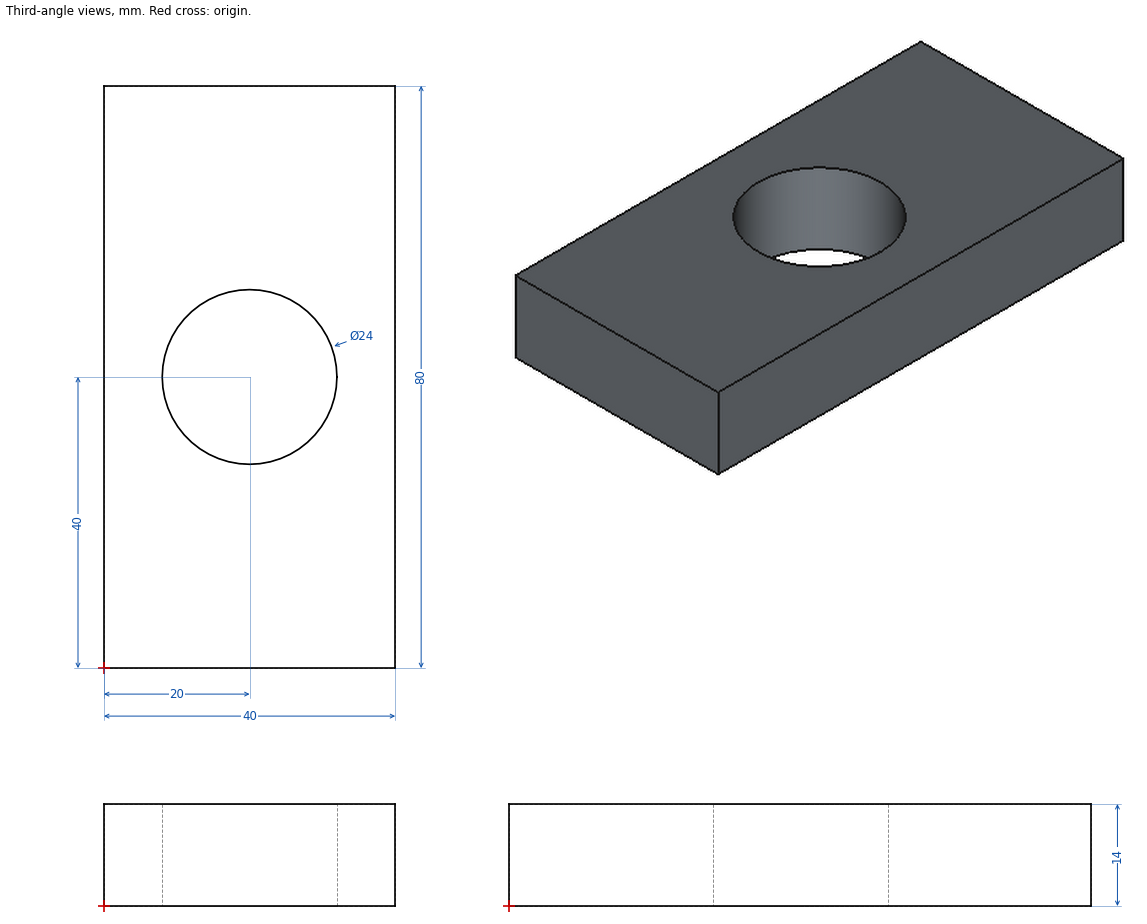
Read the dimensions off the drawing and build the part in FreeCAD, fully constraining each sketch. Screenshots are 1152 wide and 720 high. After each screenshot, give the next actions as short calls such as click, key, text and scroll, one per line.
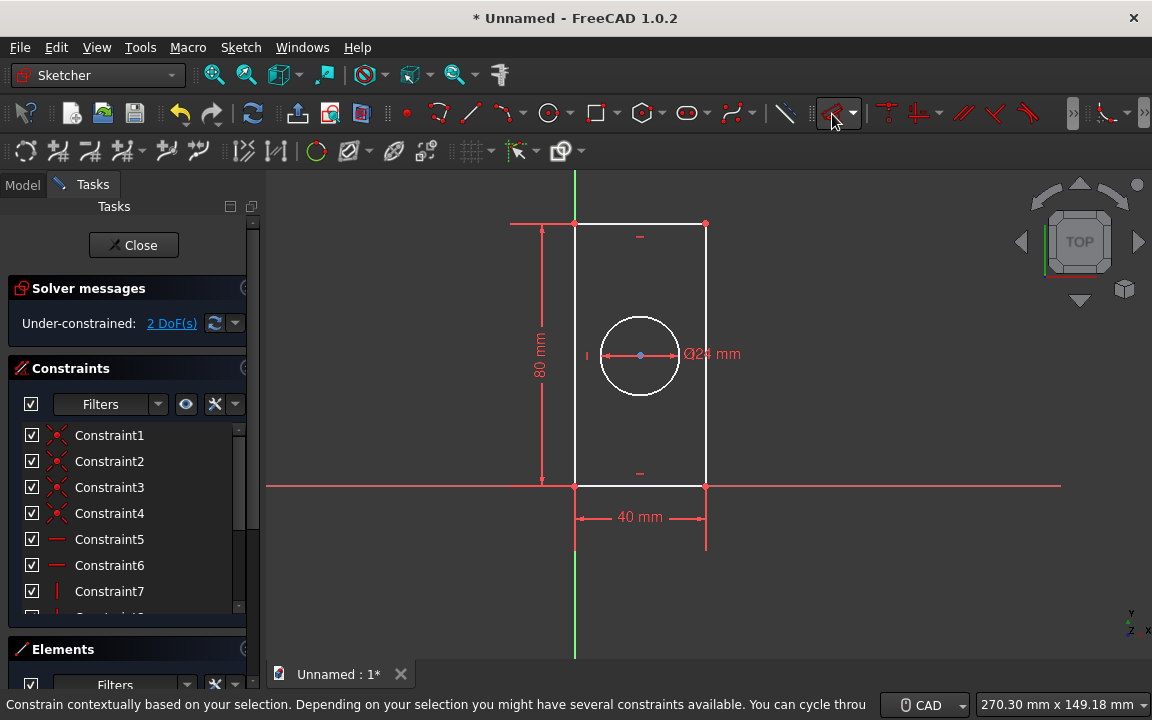
click(640, 356)
click(607, 520)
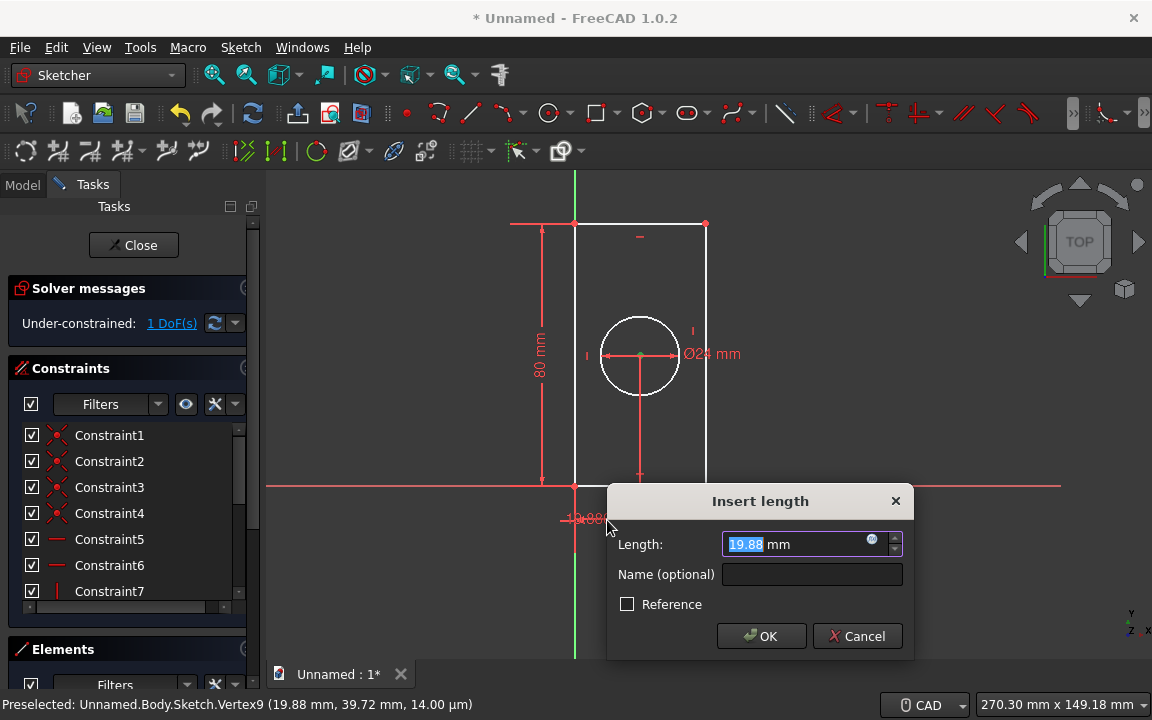
text(20)
key(Return)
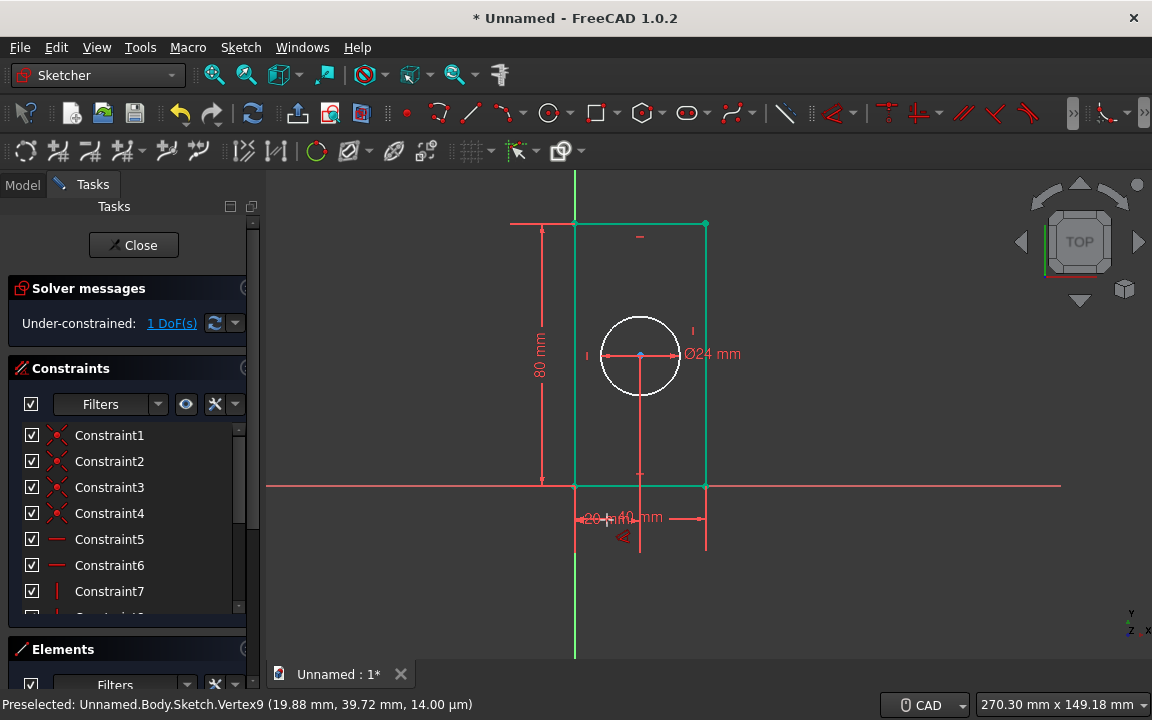
click(640, 356)
click(541, 421)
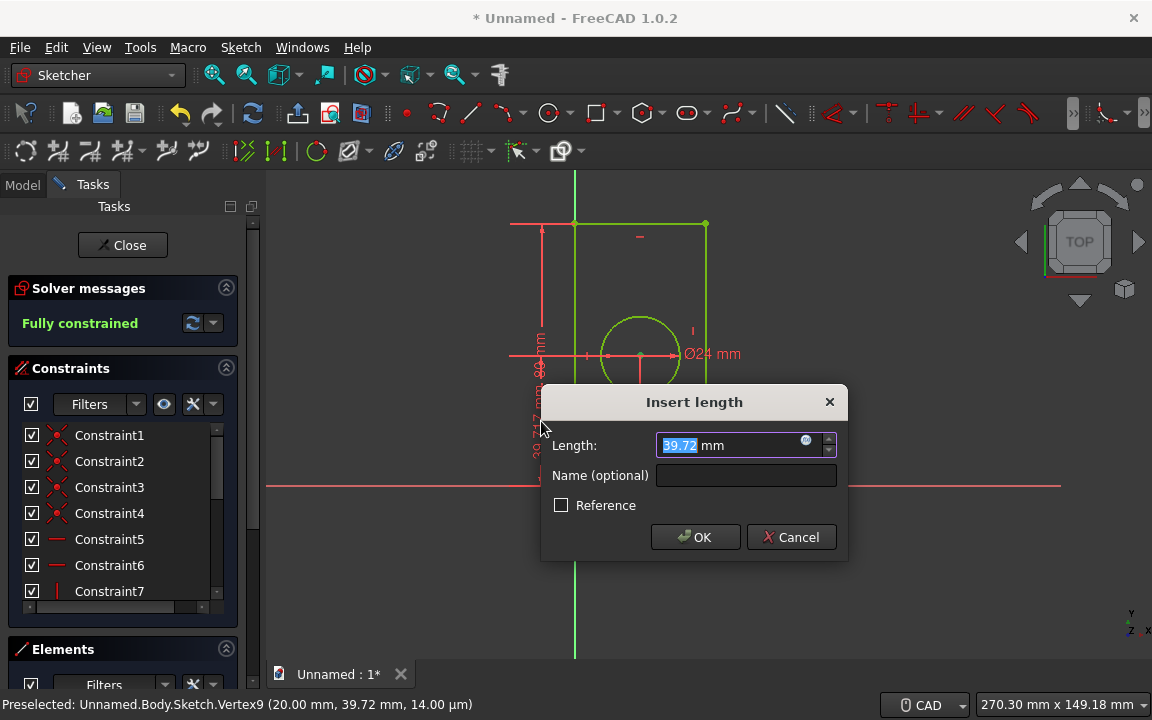
text(40)
key(Return)
key(Escape)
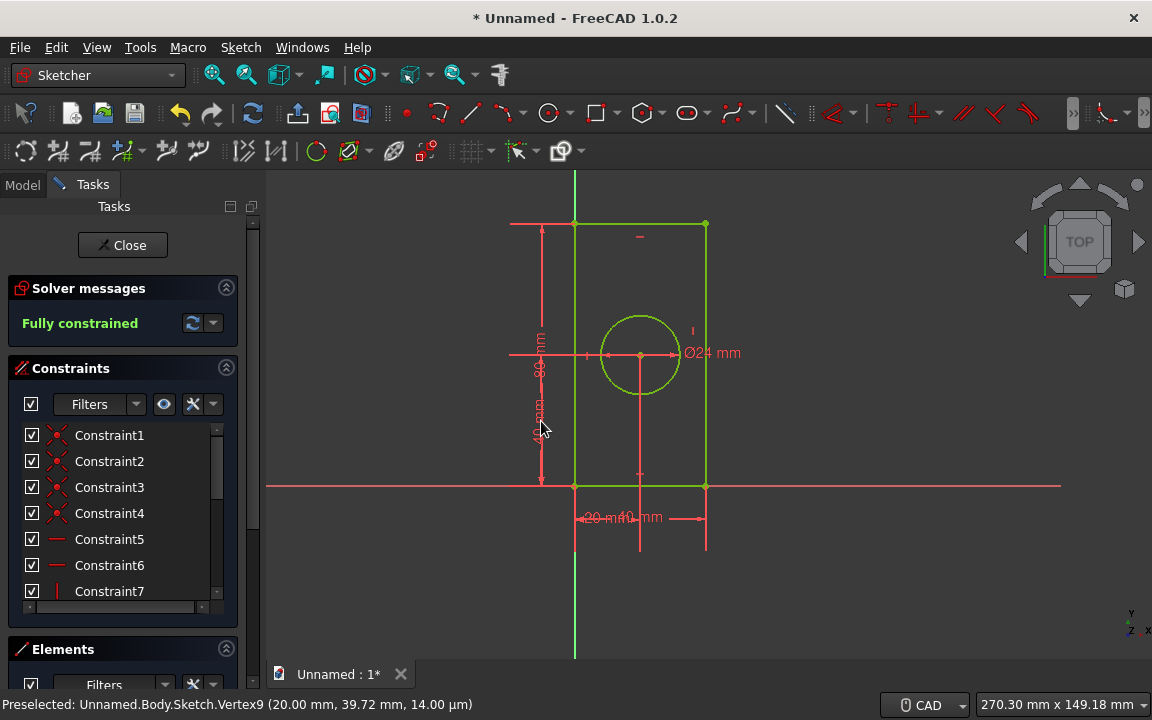
click(123, 245)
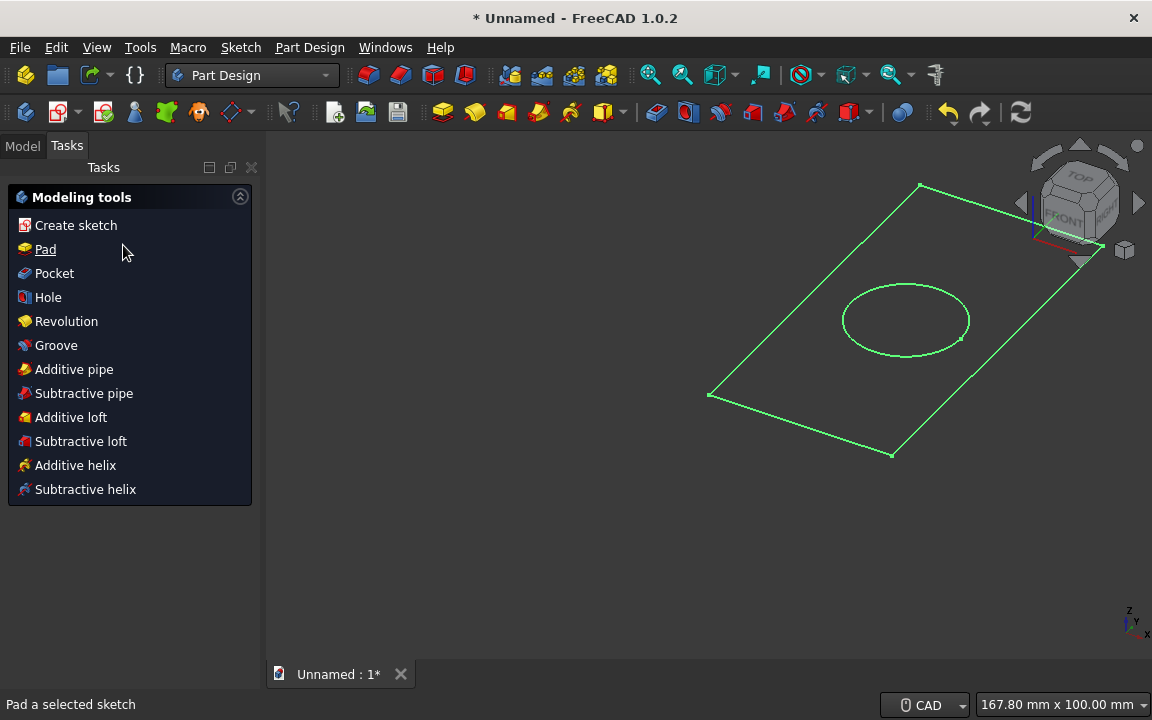
click(444, 112)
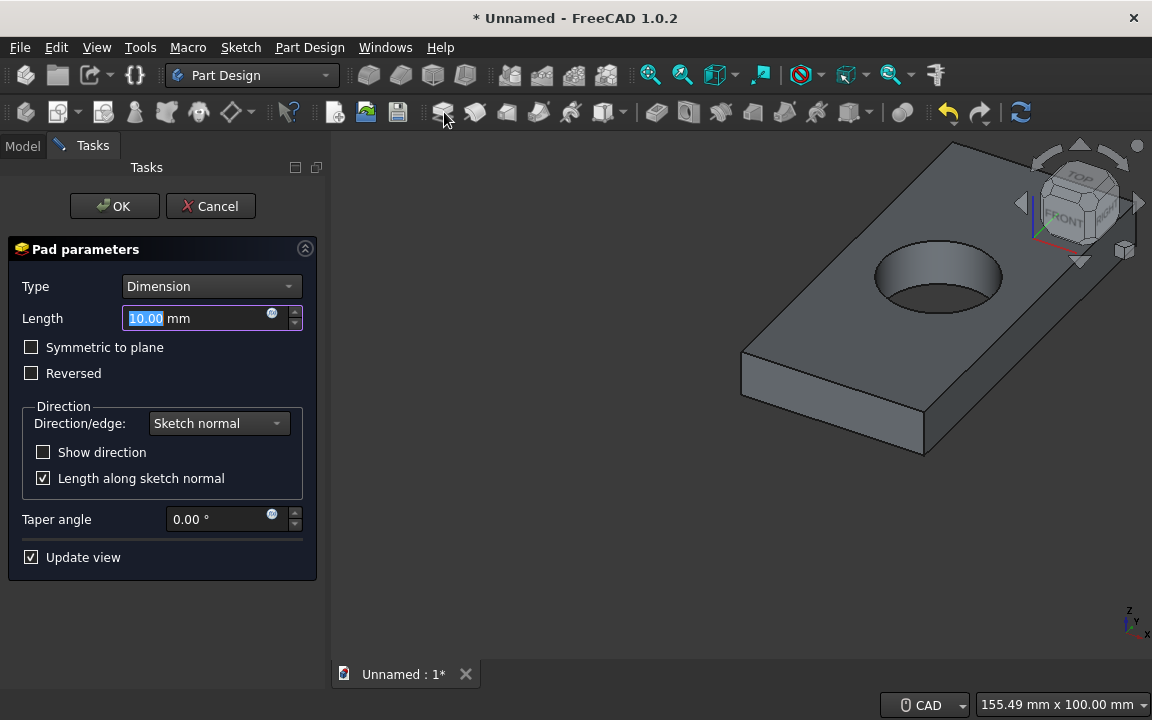
text(14)
key(Tab)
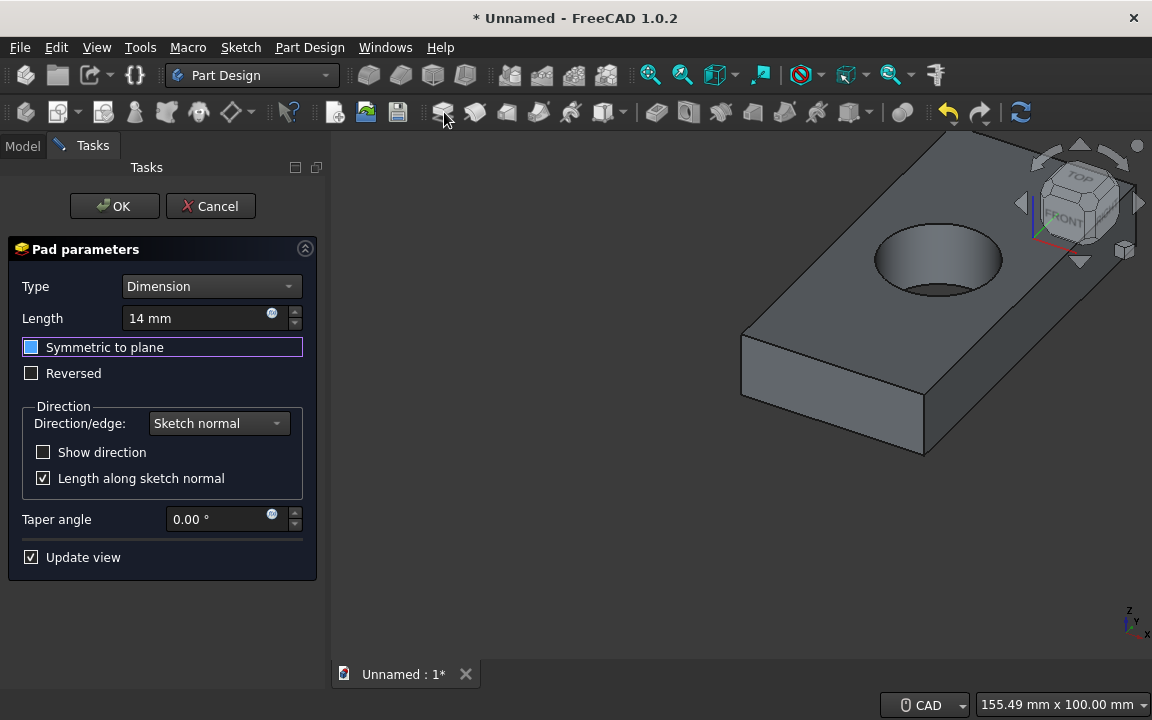
click(115, 206)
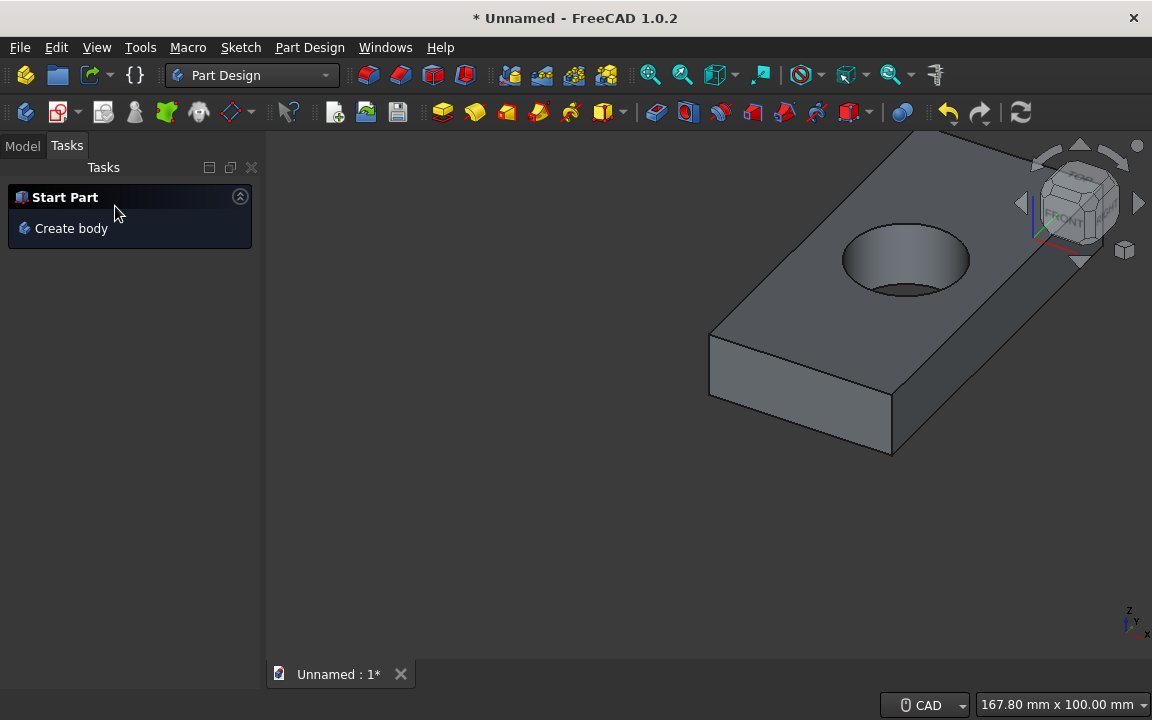
key(0)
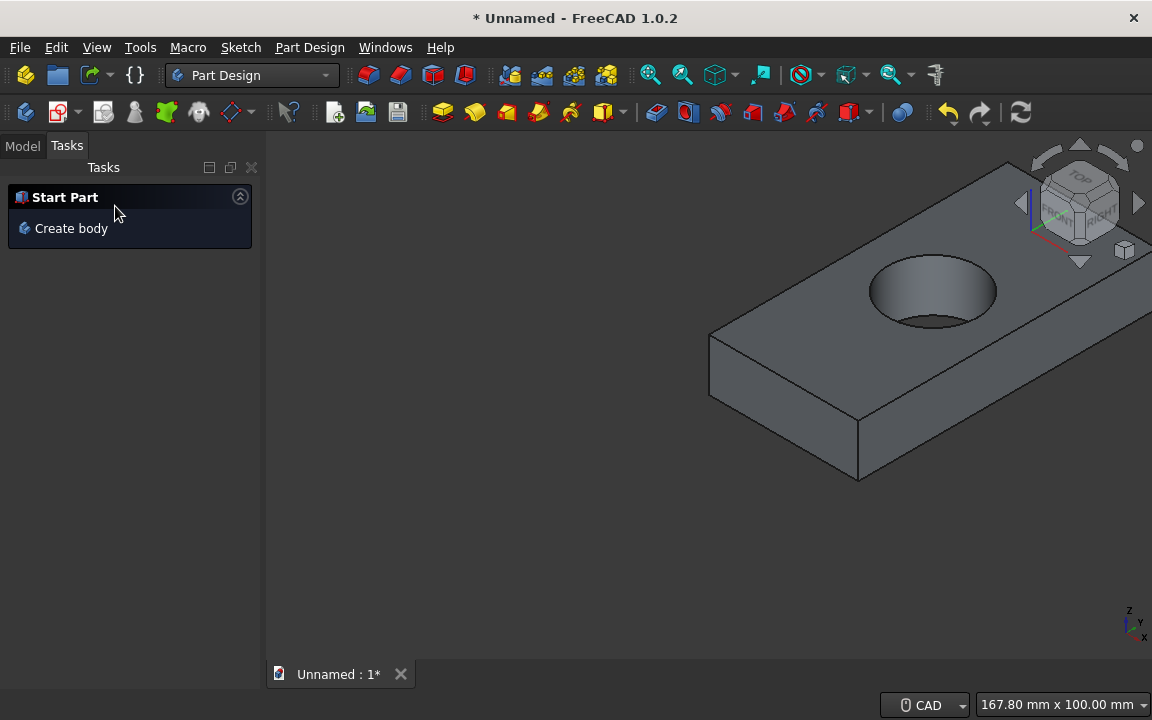
click(652, 76)